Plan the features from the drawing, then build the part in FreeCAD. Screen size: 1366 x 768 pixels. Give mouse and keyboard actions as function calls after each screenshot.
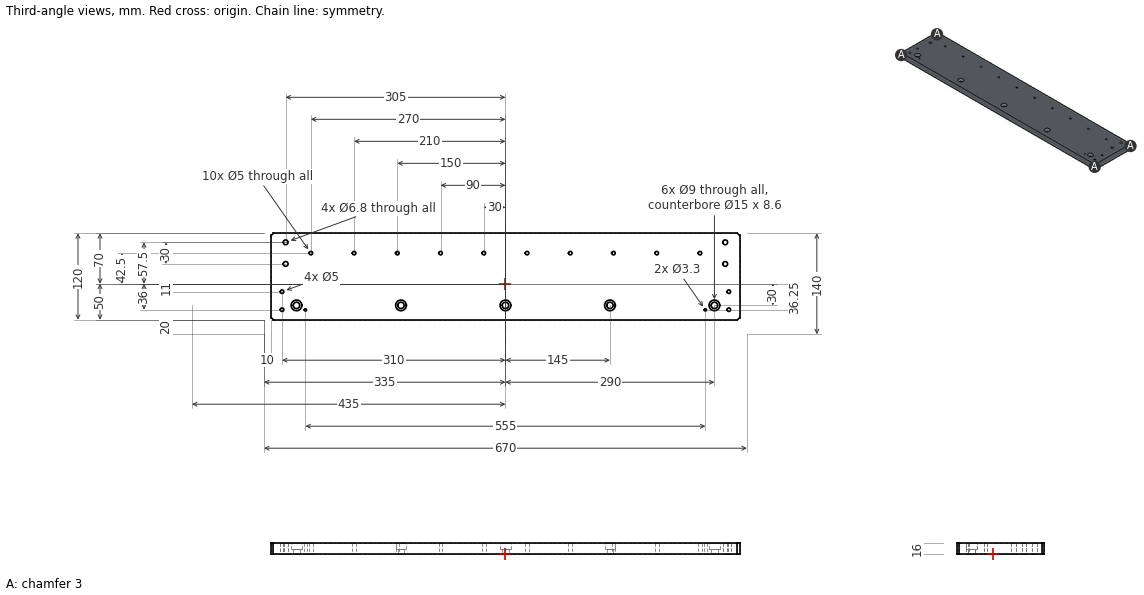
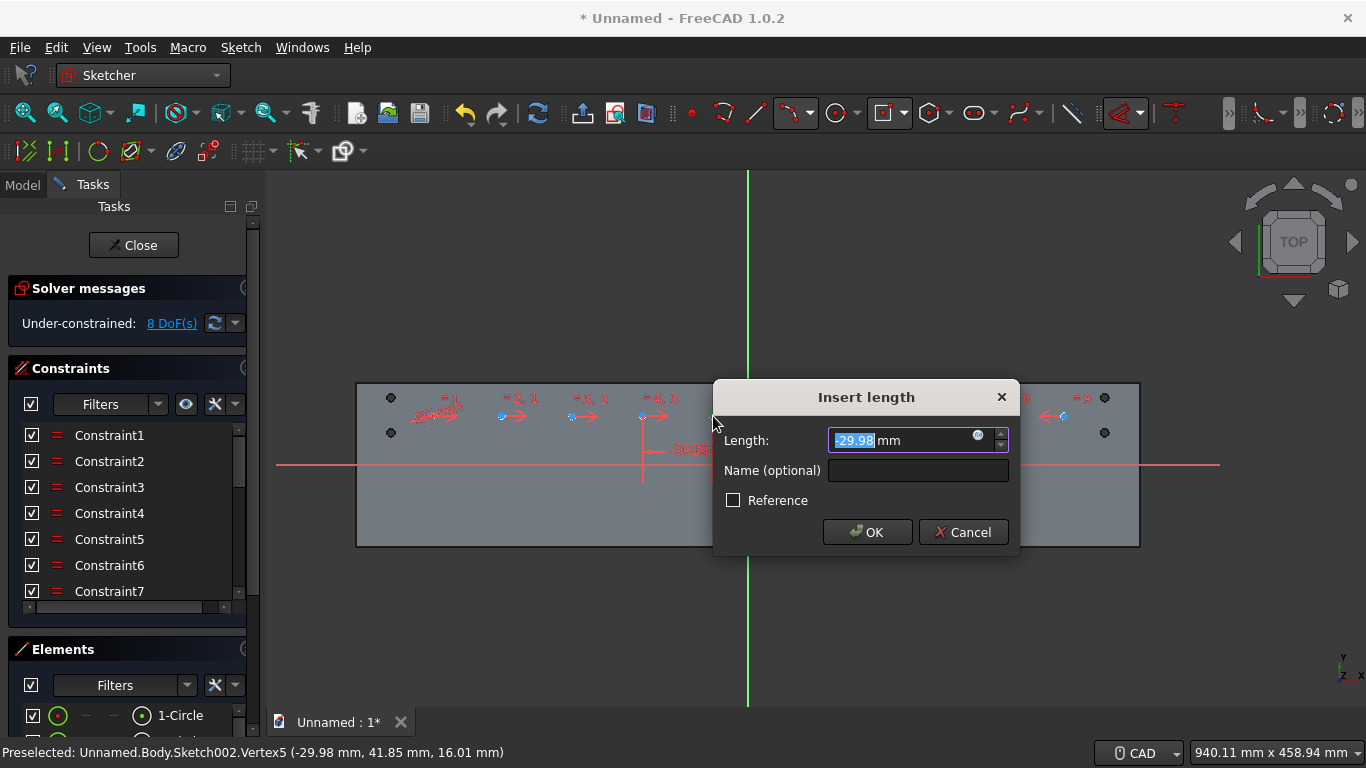
text(-30)
key(Return)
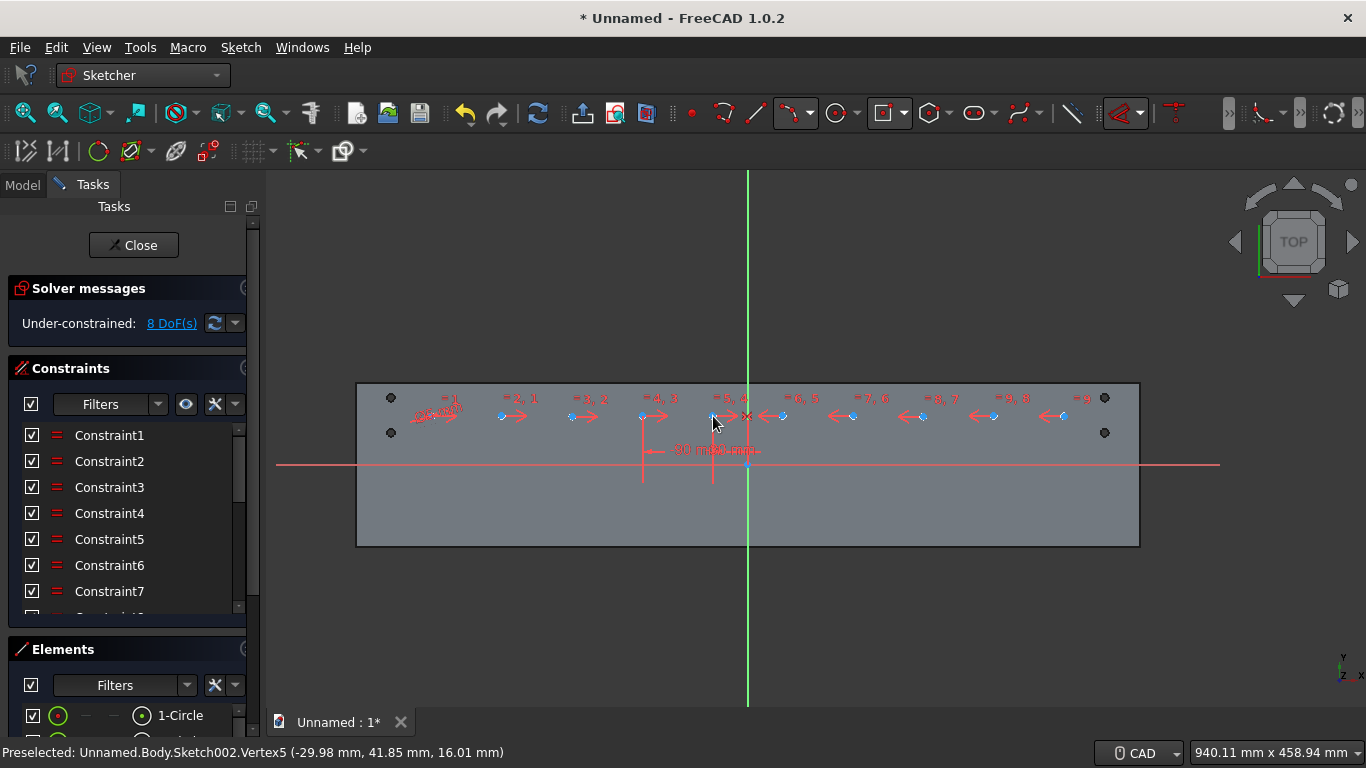
click(432, 416)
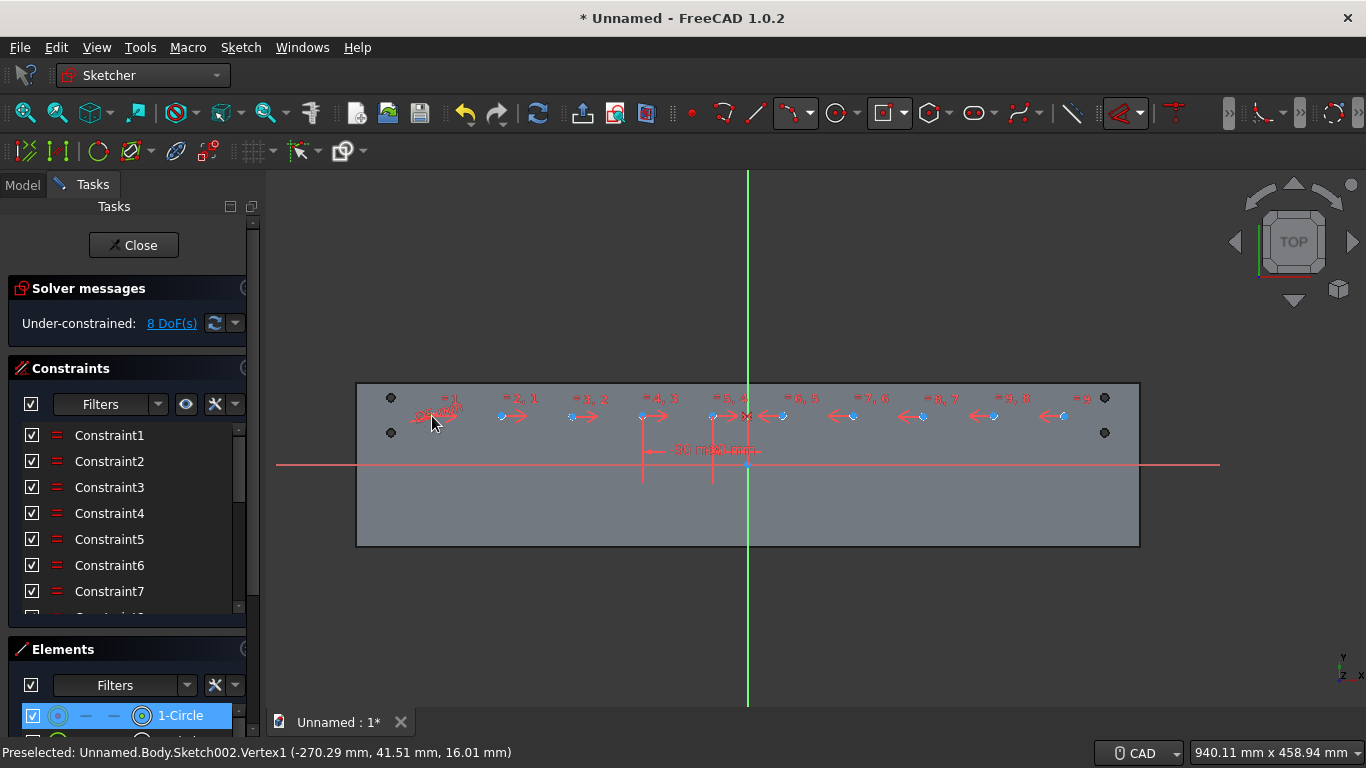
click(1142, 114)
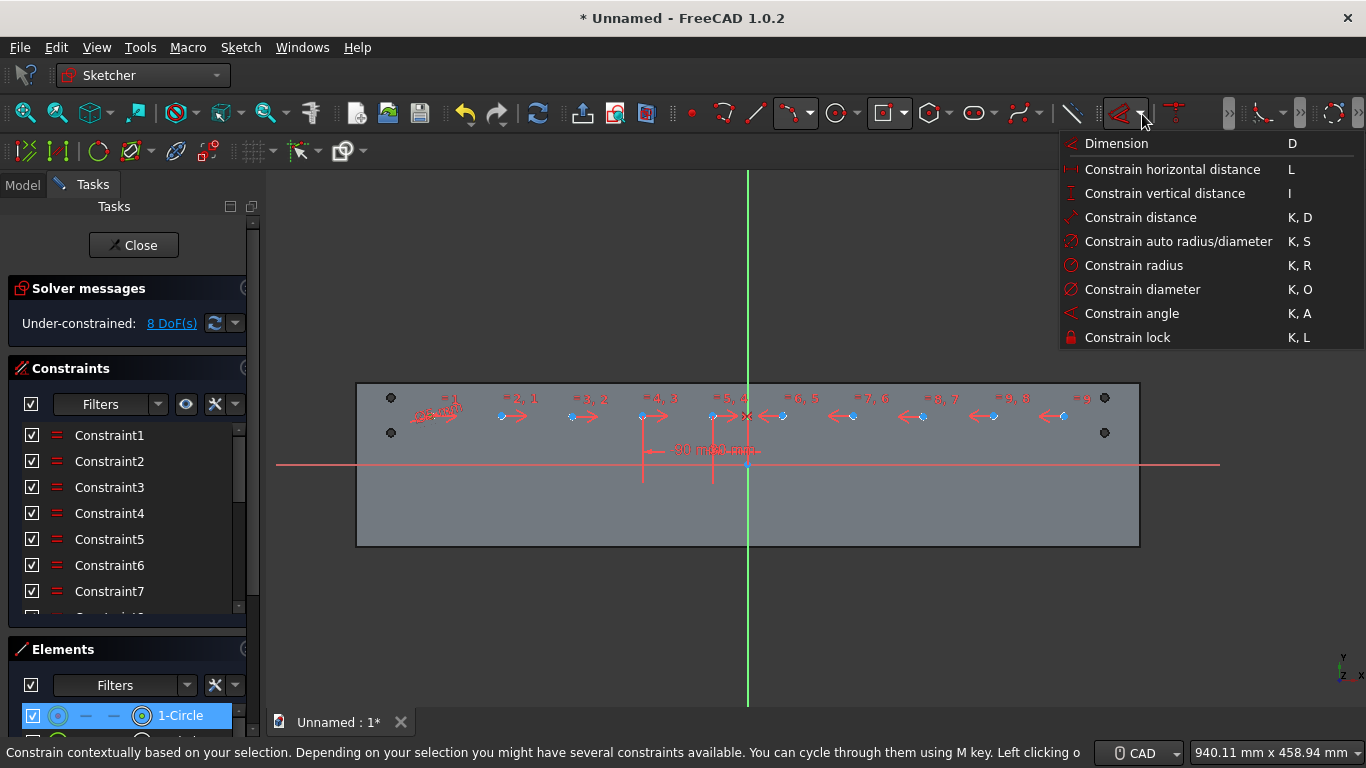
click(1212, 169)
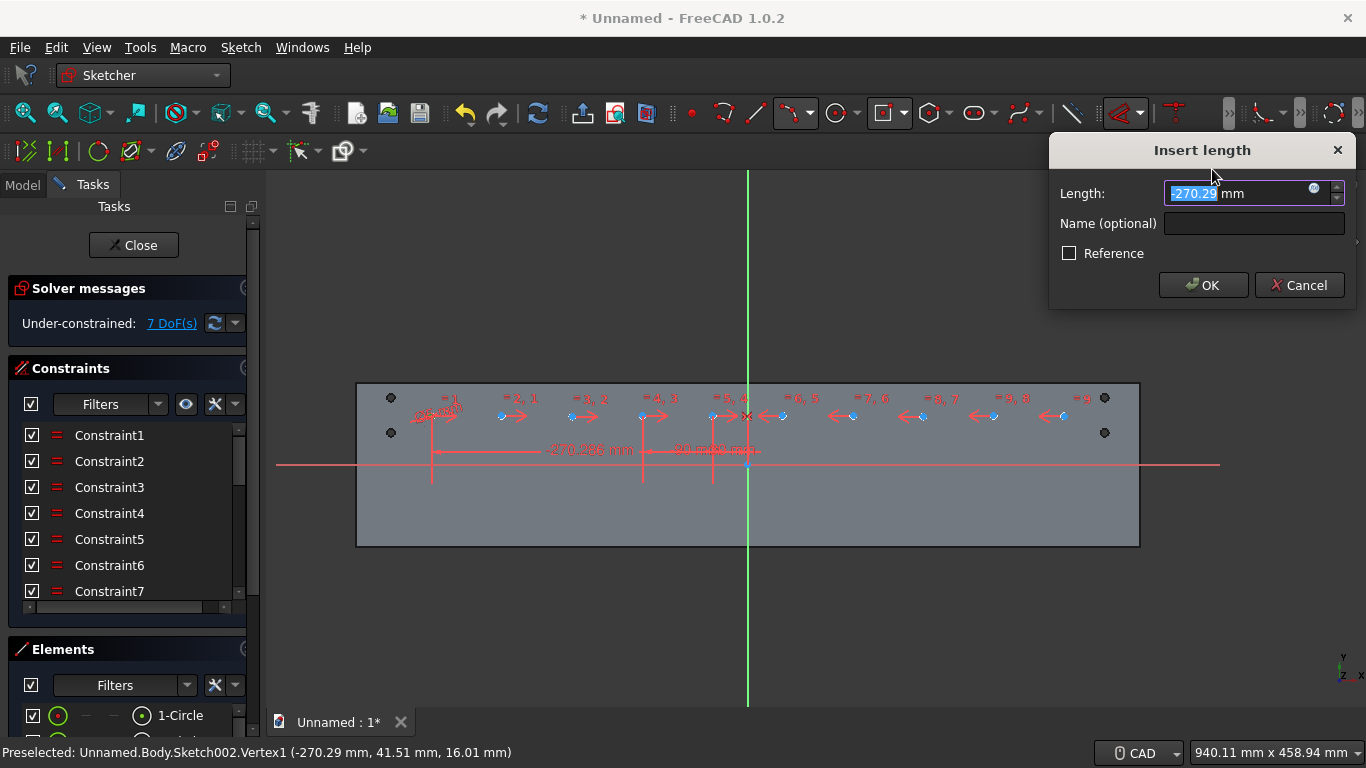
text(-270)
key(Return)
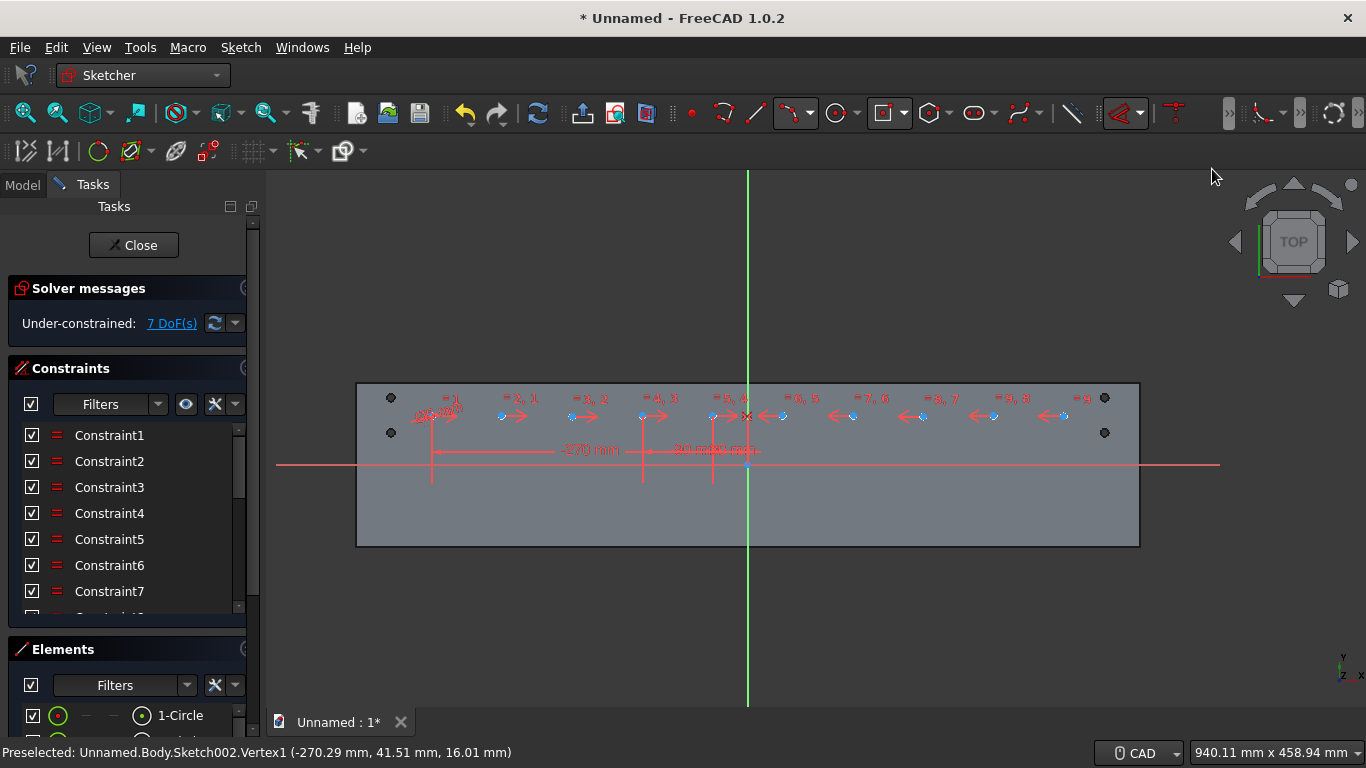
click(502, 416)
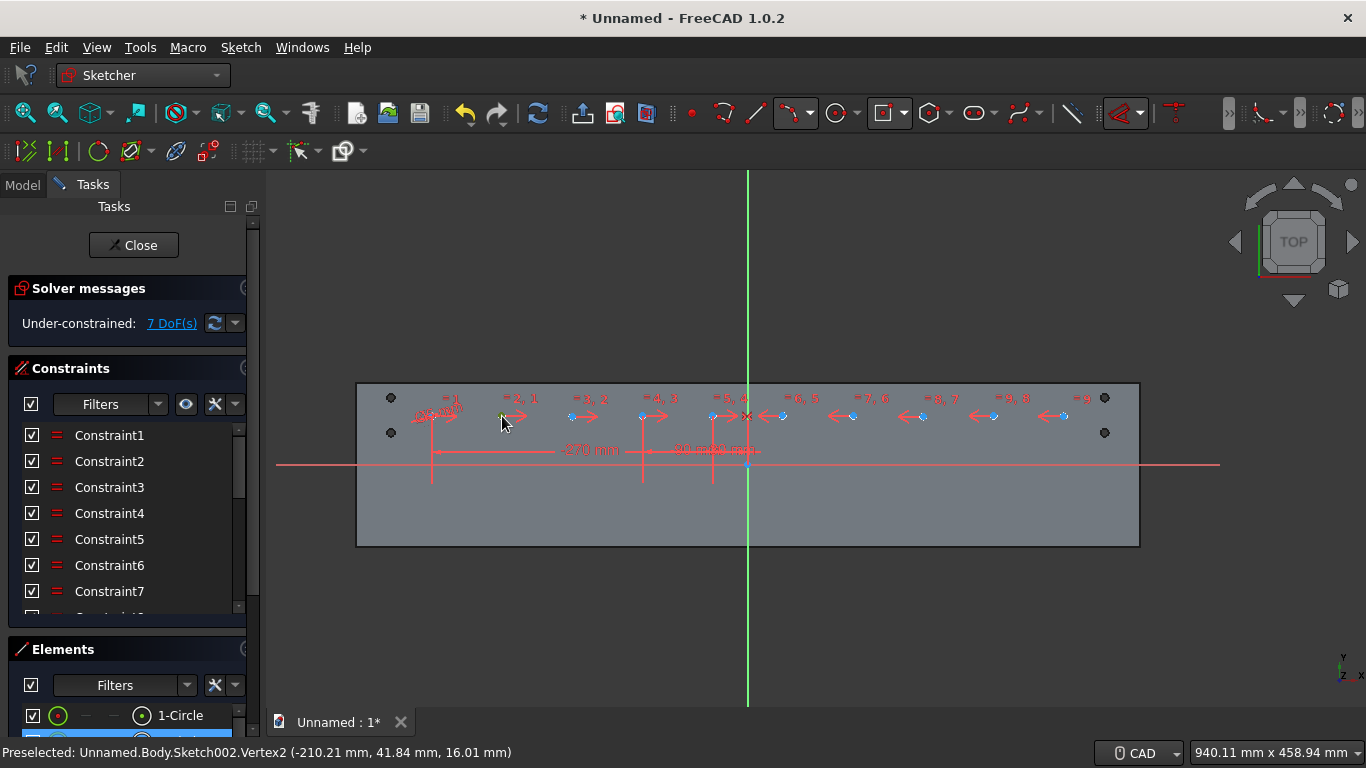
click(1142, 114)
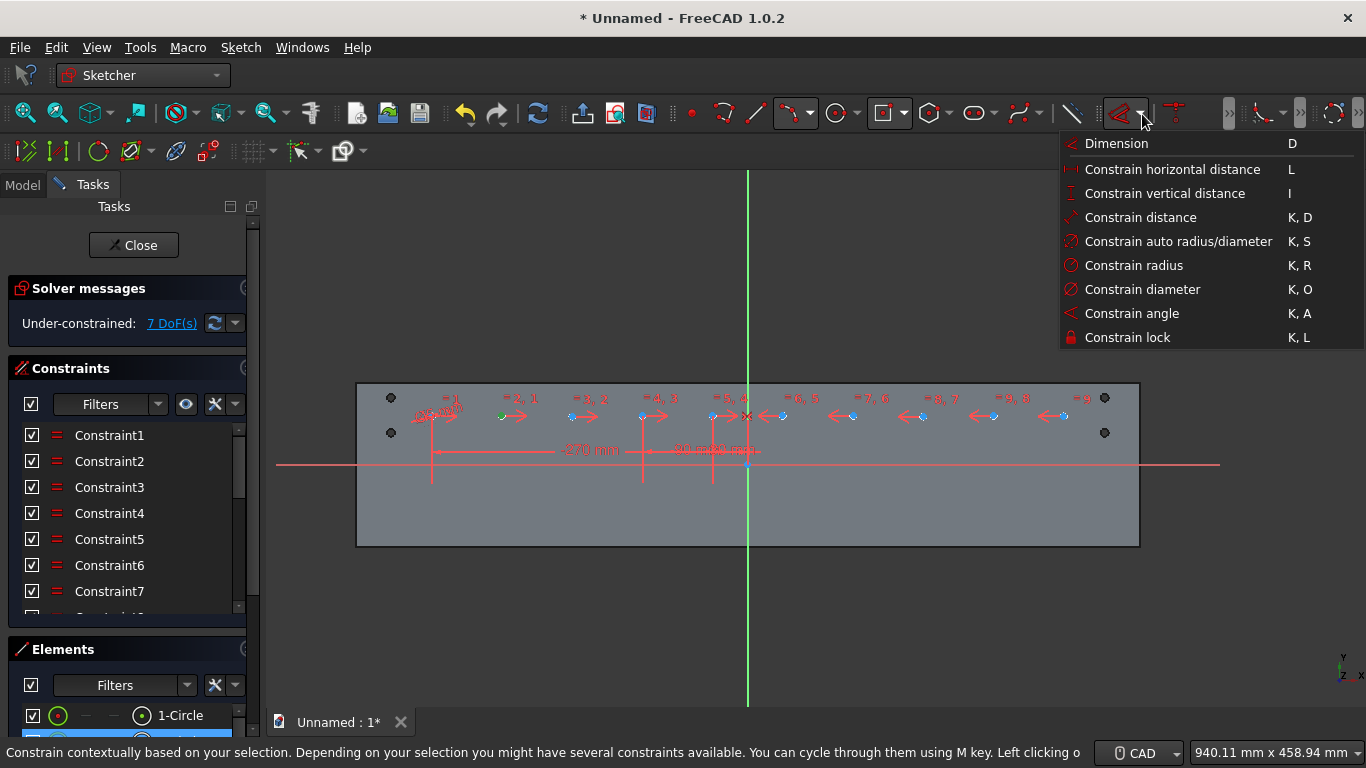
click(1212, 169)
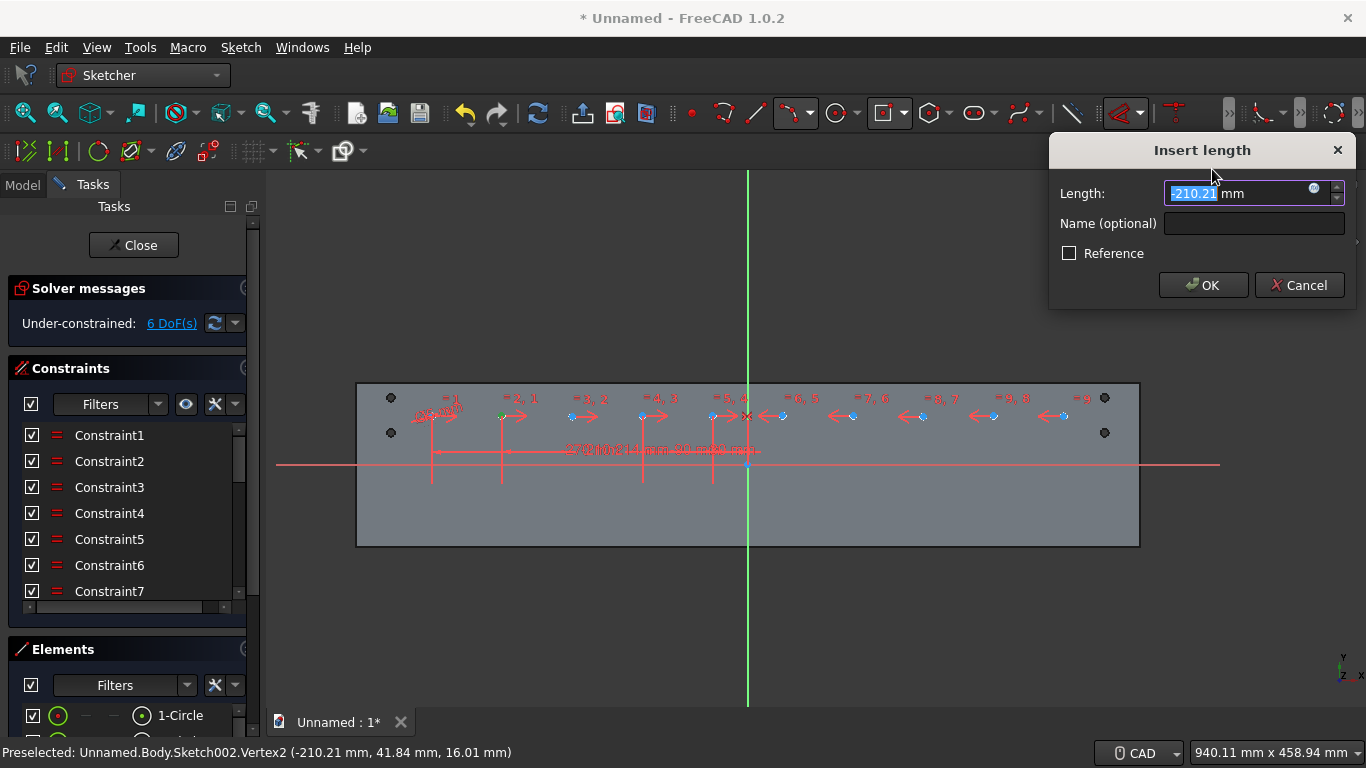
text(-210)
key(Return)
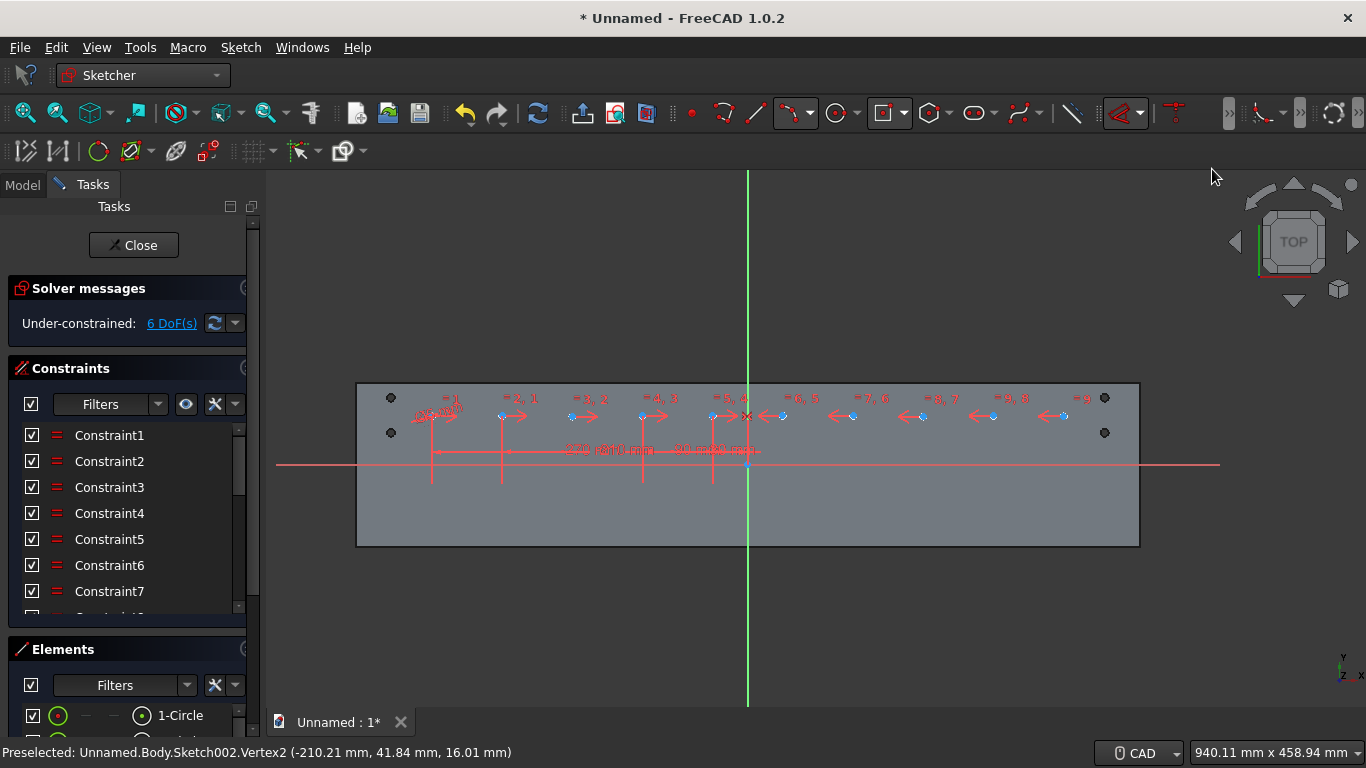
click(572, 417)